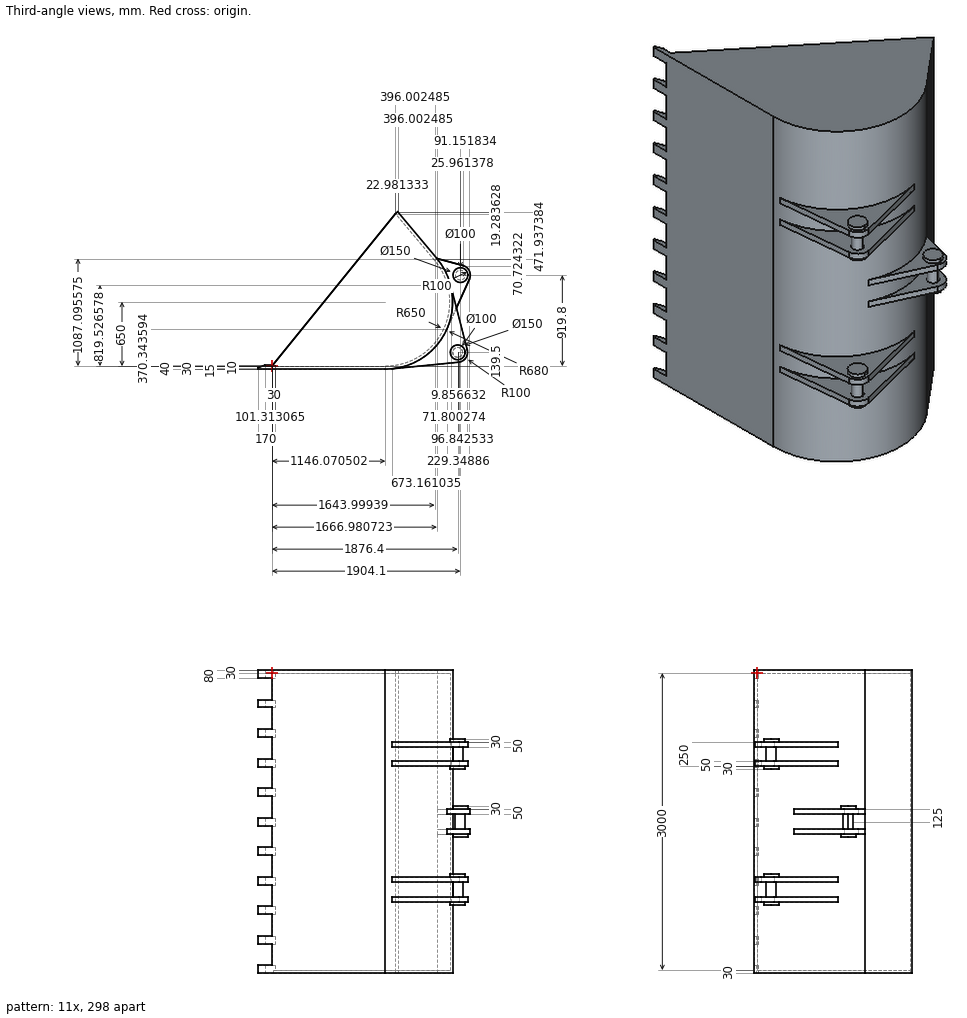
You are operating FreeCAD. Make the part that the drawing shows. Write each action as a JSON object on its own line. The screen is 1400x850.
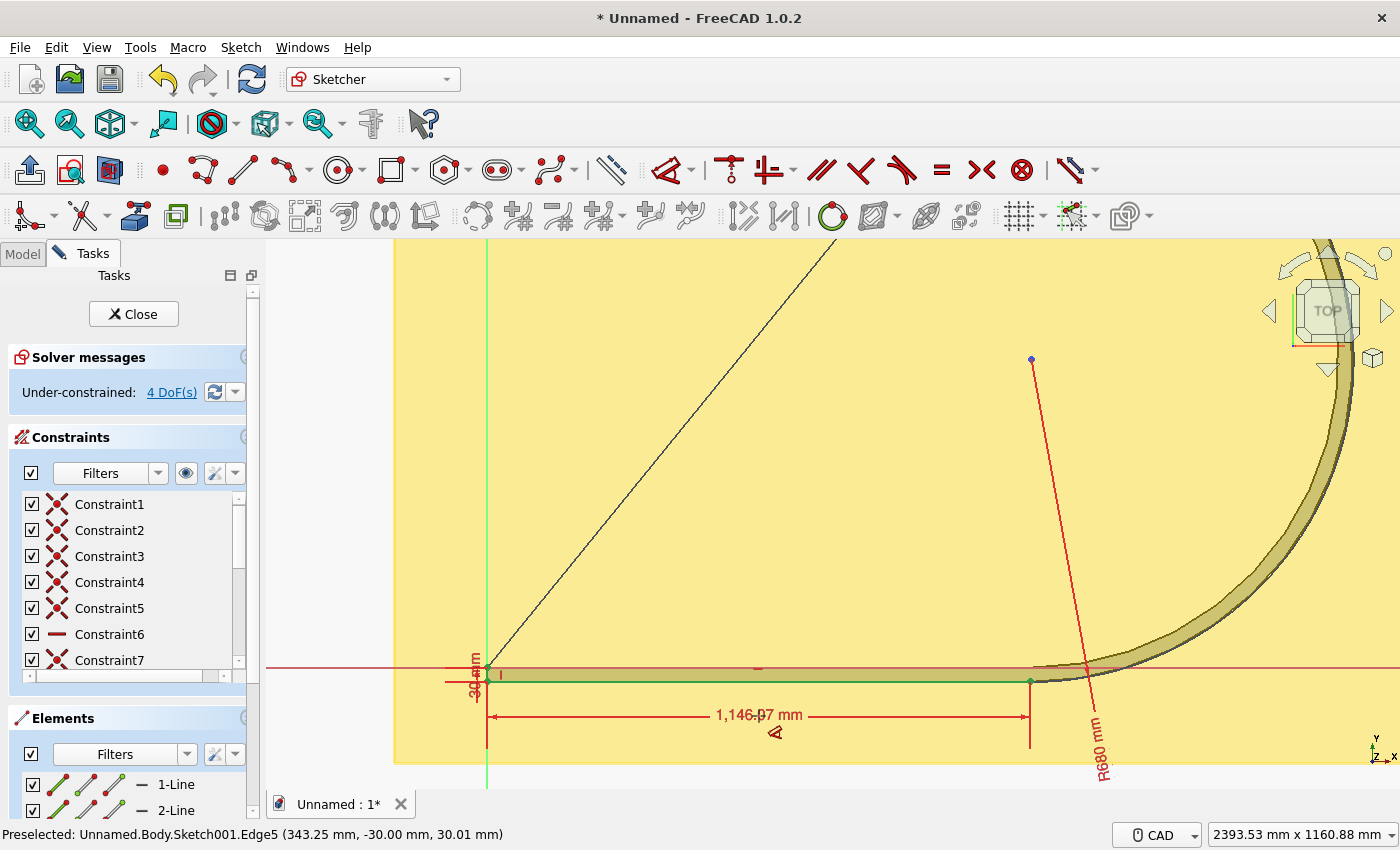
{"action": "scroll", "coordinate": [650, 684], "scroll_direction": "down", "scroll_amount": 4}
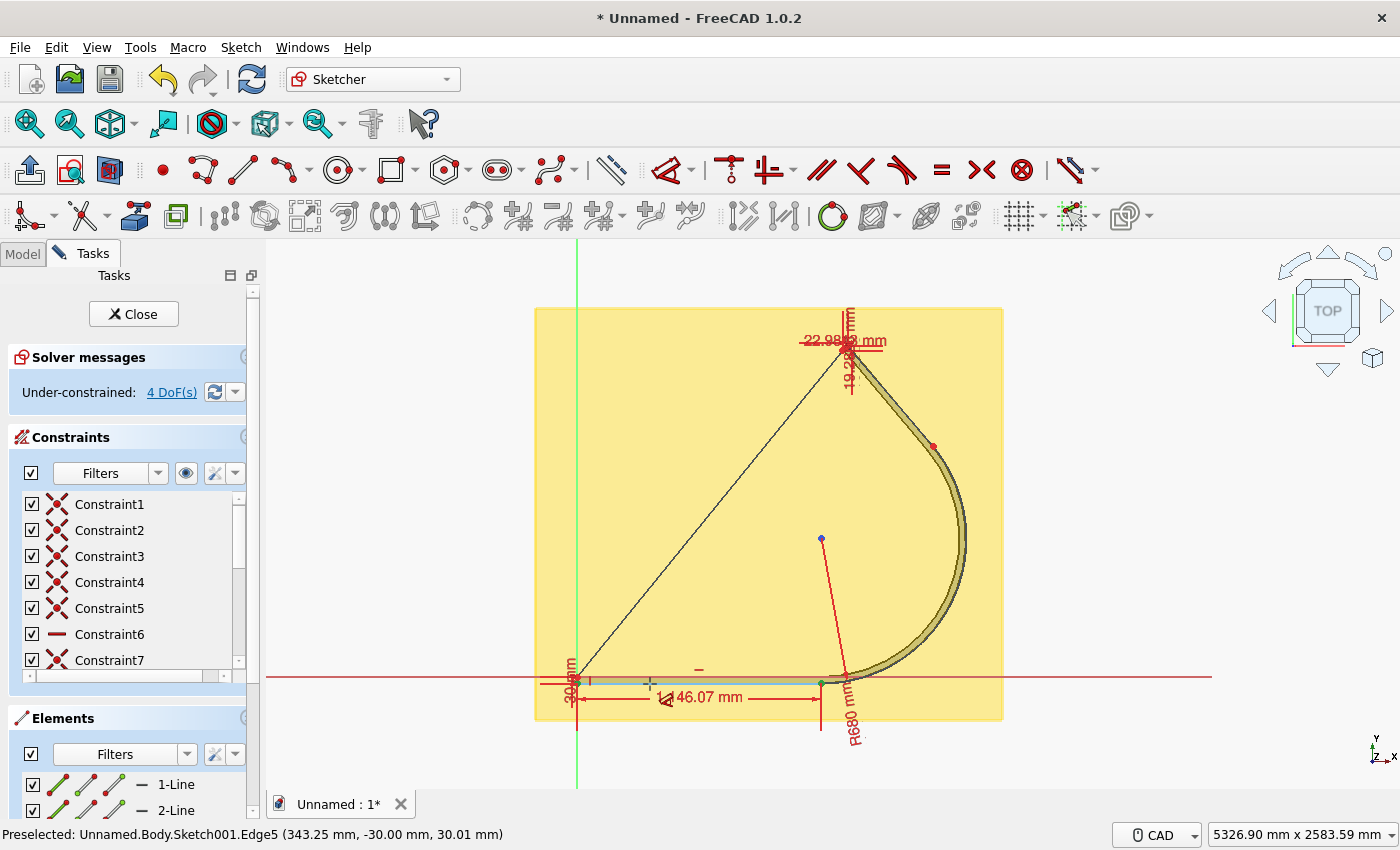
{"action": "left_click", "coordinate": [908, 417]}
{"action": "left_click", "coordinate": [891, 312]}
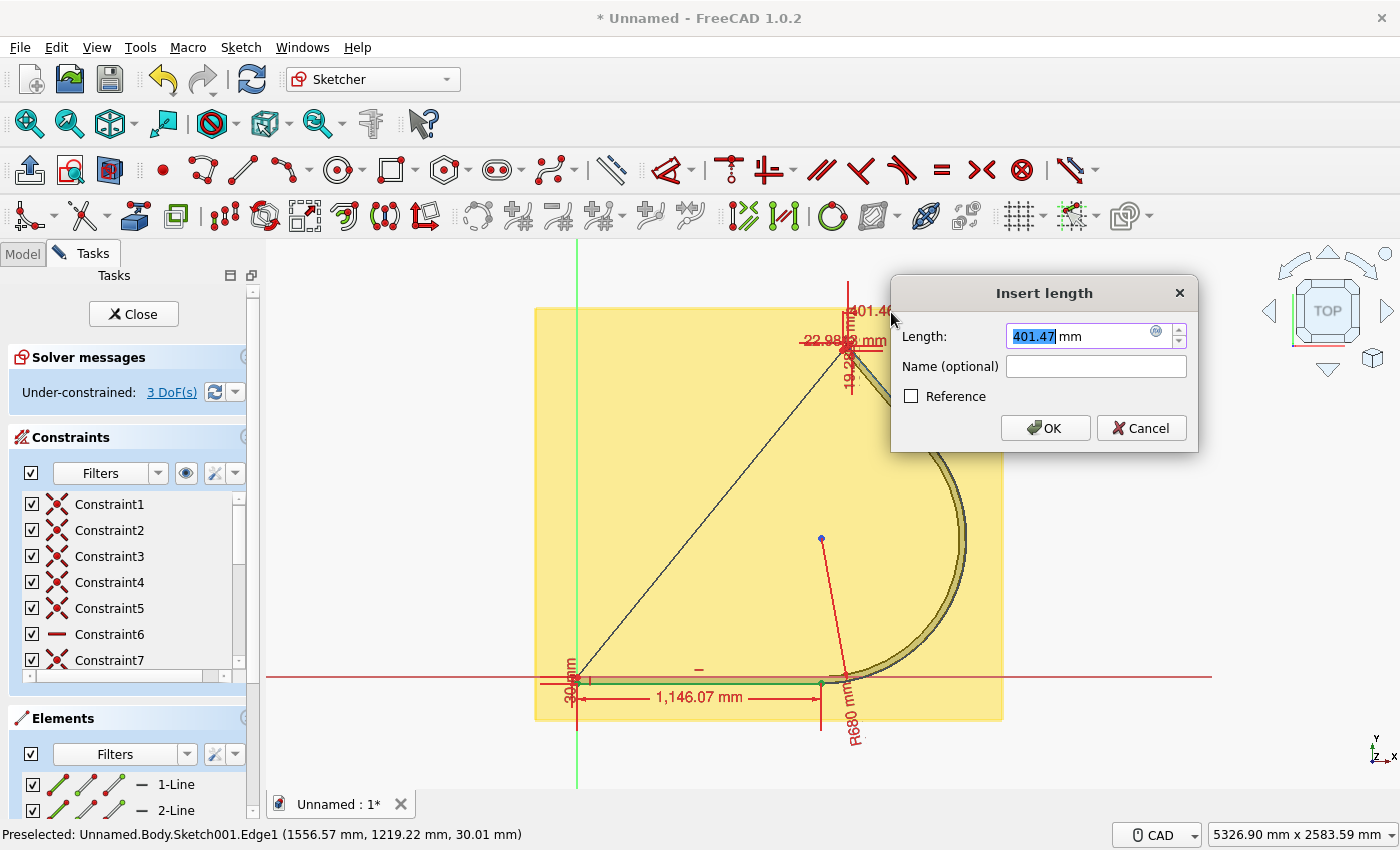
{"action": "type", "text": "396.002485"}
{"action": "key", "text": "Return"}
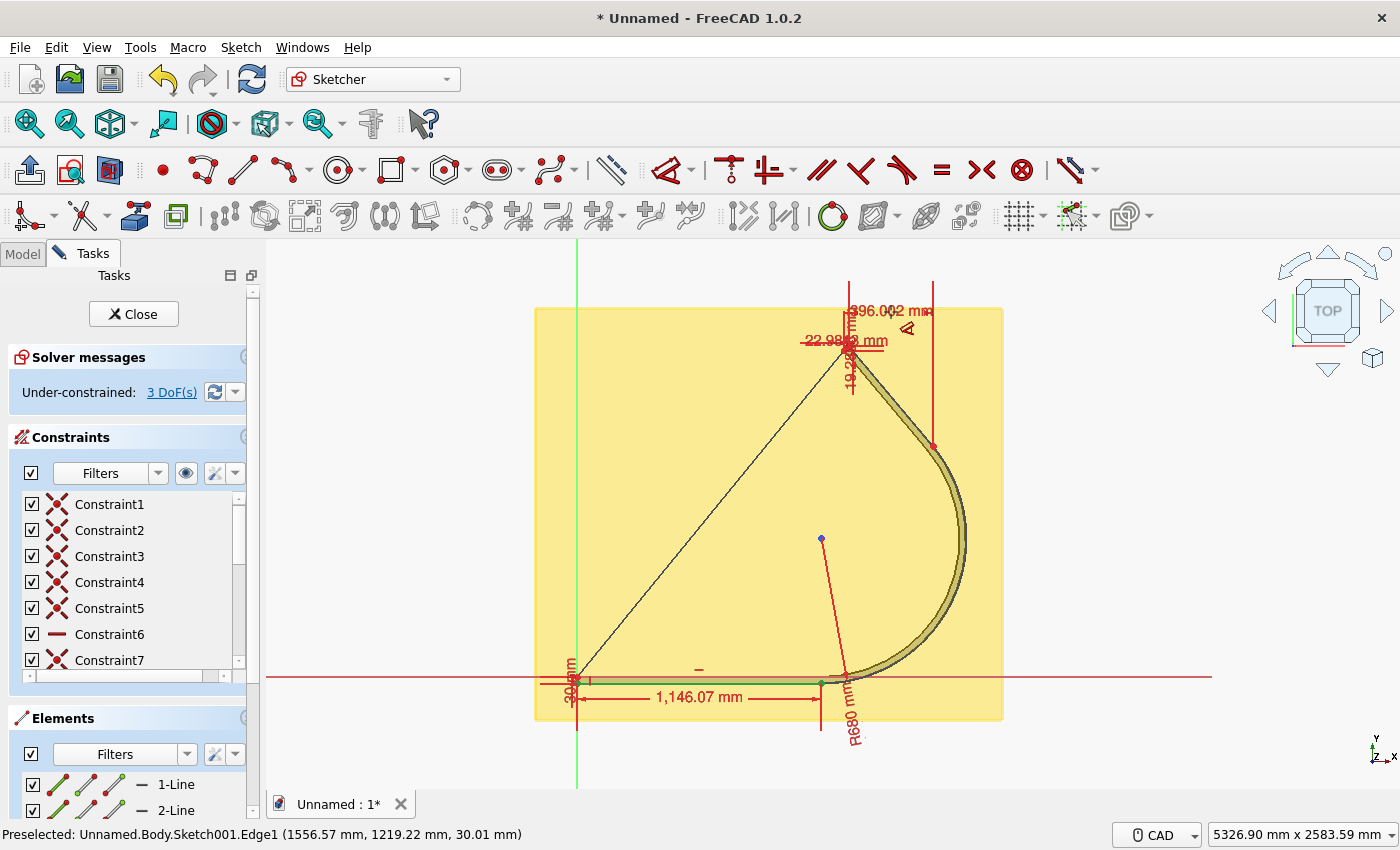
{"action": "left_click", "coordinate": [908, 417]}
{"action": "left_click", "coordinate": [967, 397]}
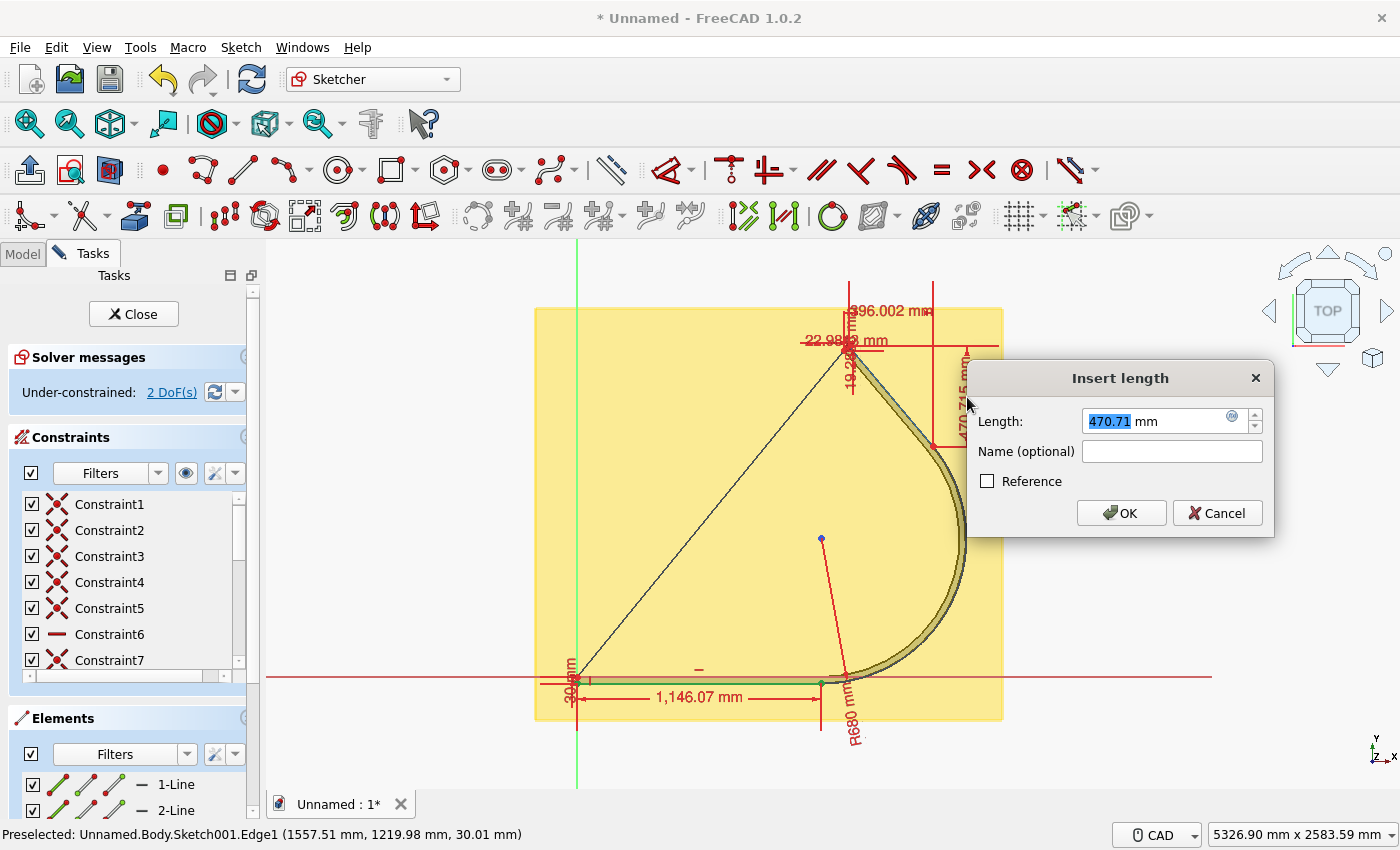
{"action": "type", "text": "471.937384"}
{"action": "key", "text": "Return"}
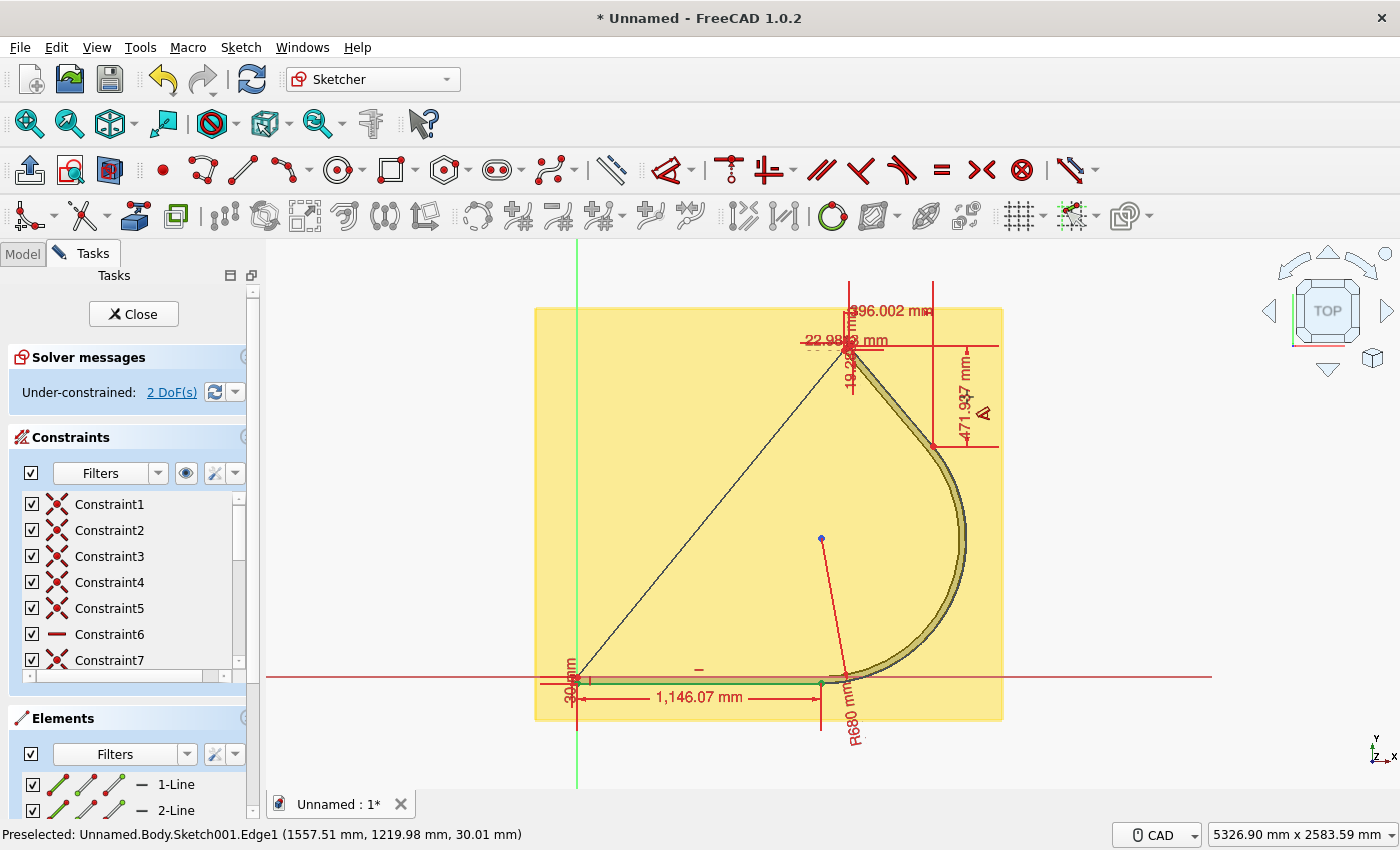
{"action": "left_click", "coordinate": [933, 447]}
{"action": "left_click", "coordinate": [755, 413]}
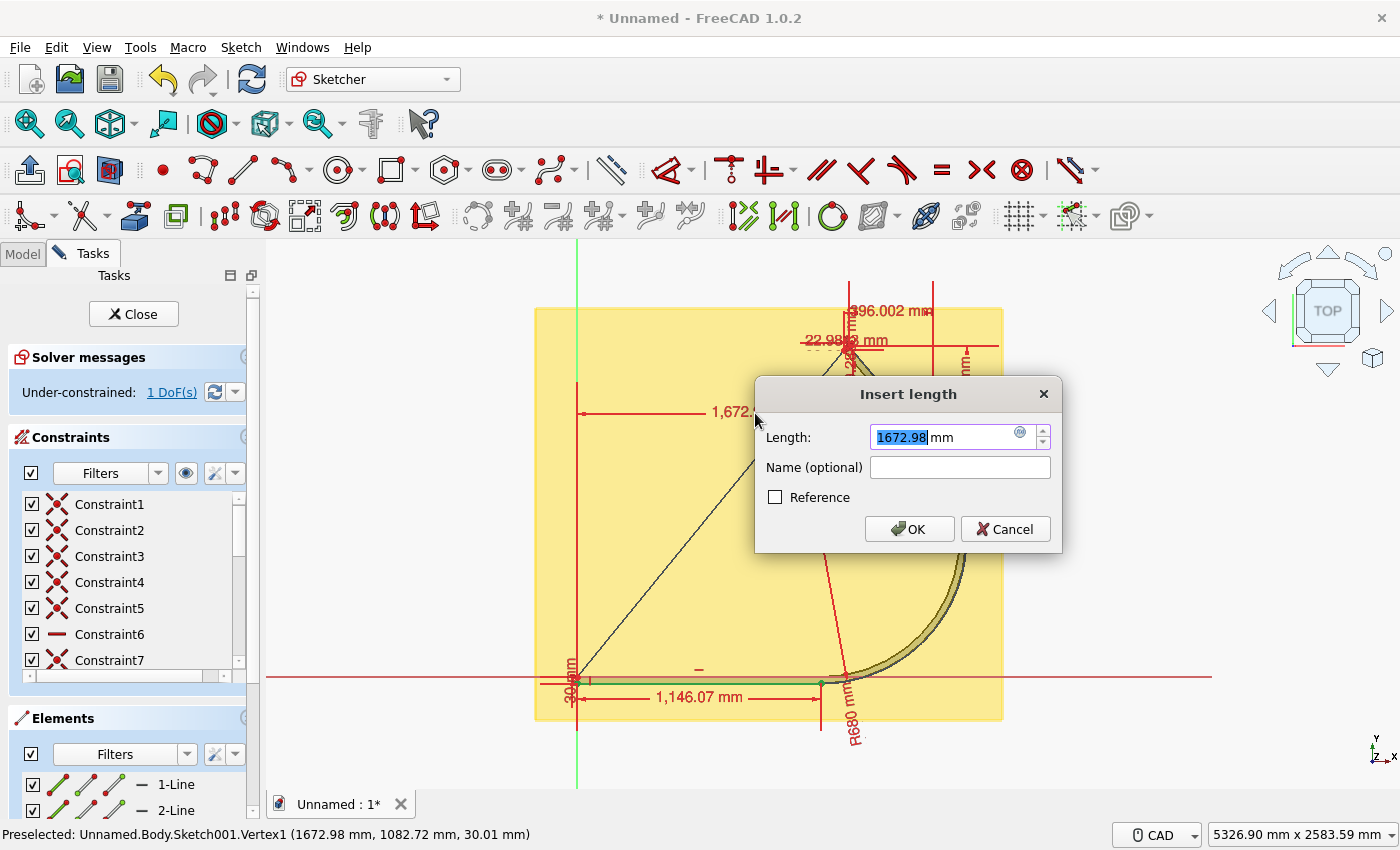
{"action": "type", "text": "1666.980723"}
{"action": "key", "text": "Return"}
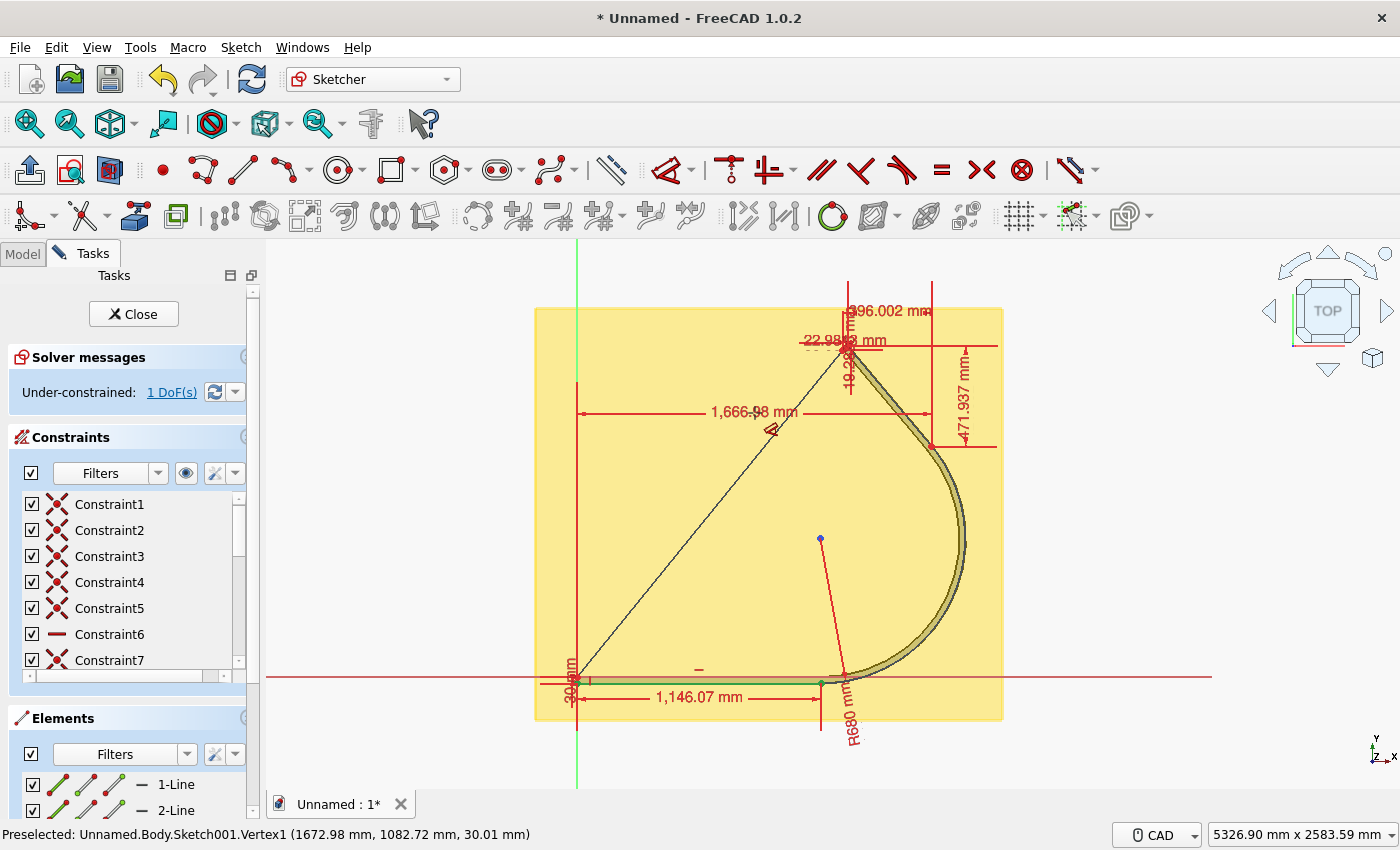
{"action": "left_click", "coordinate": [932, 447]}
{"action": "left_click", "coordinate": [543, 562]}